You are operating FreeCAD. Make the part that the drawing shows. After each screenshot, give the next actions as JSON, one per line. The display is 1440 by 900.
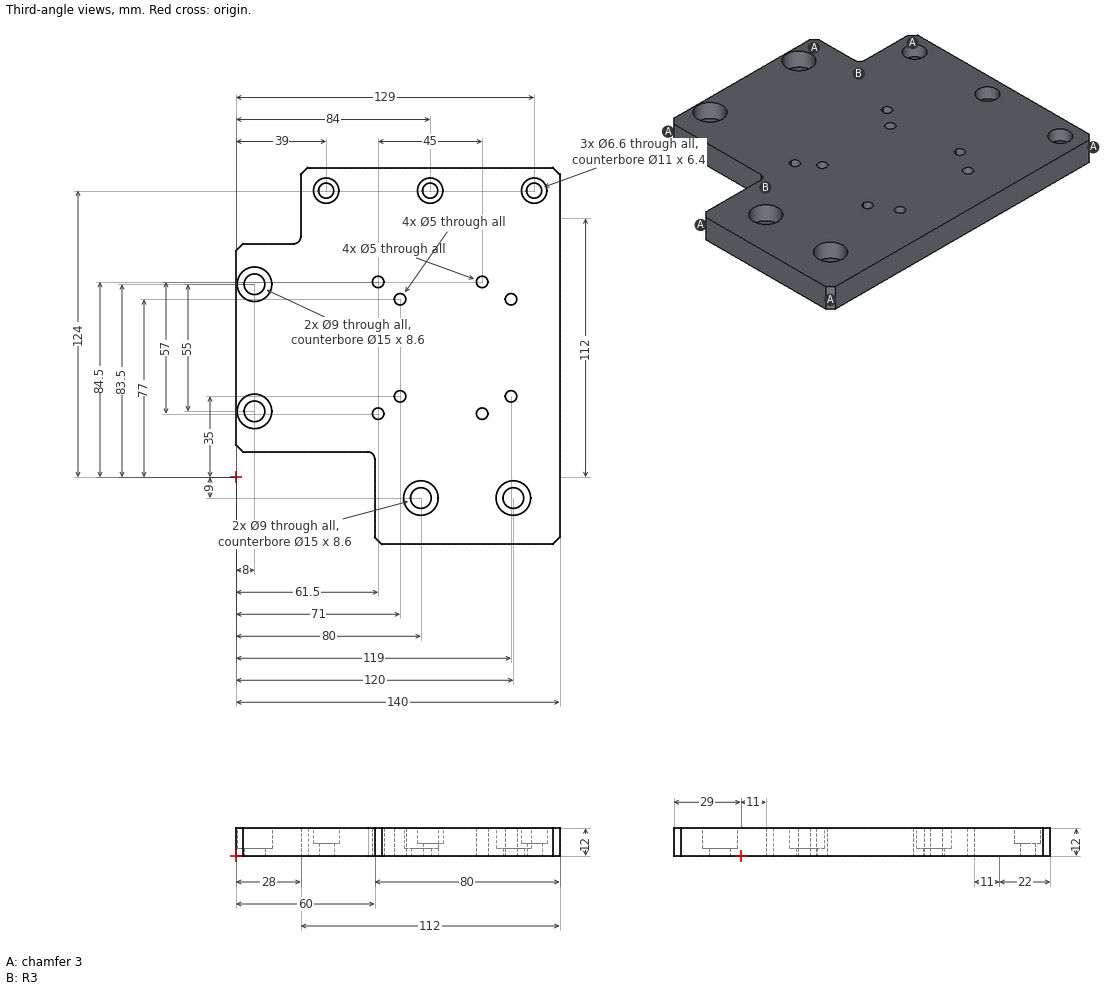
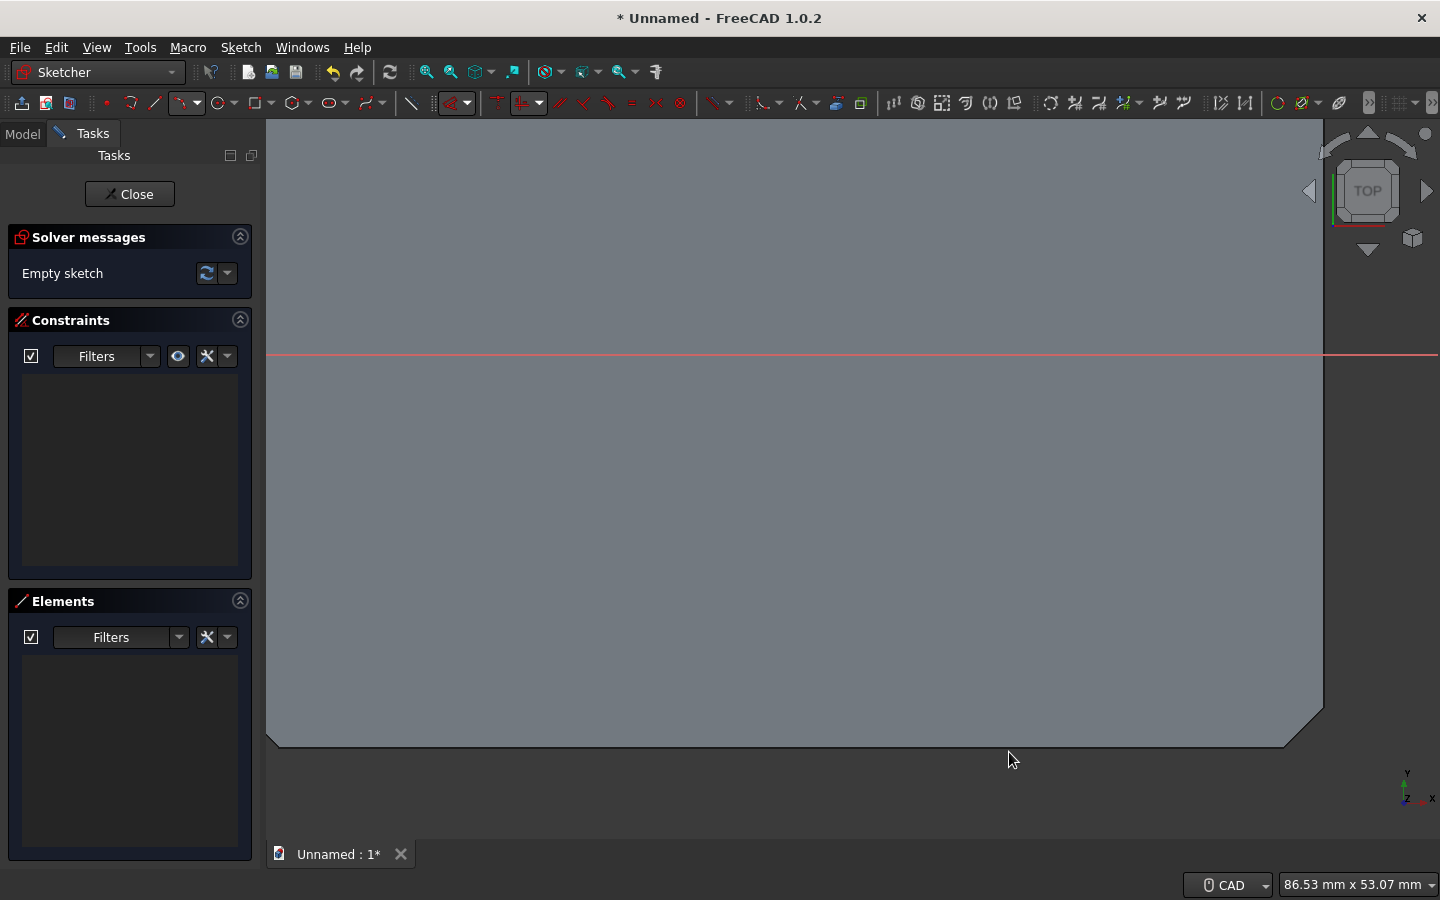
{"action": "key", "text": "g c"}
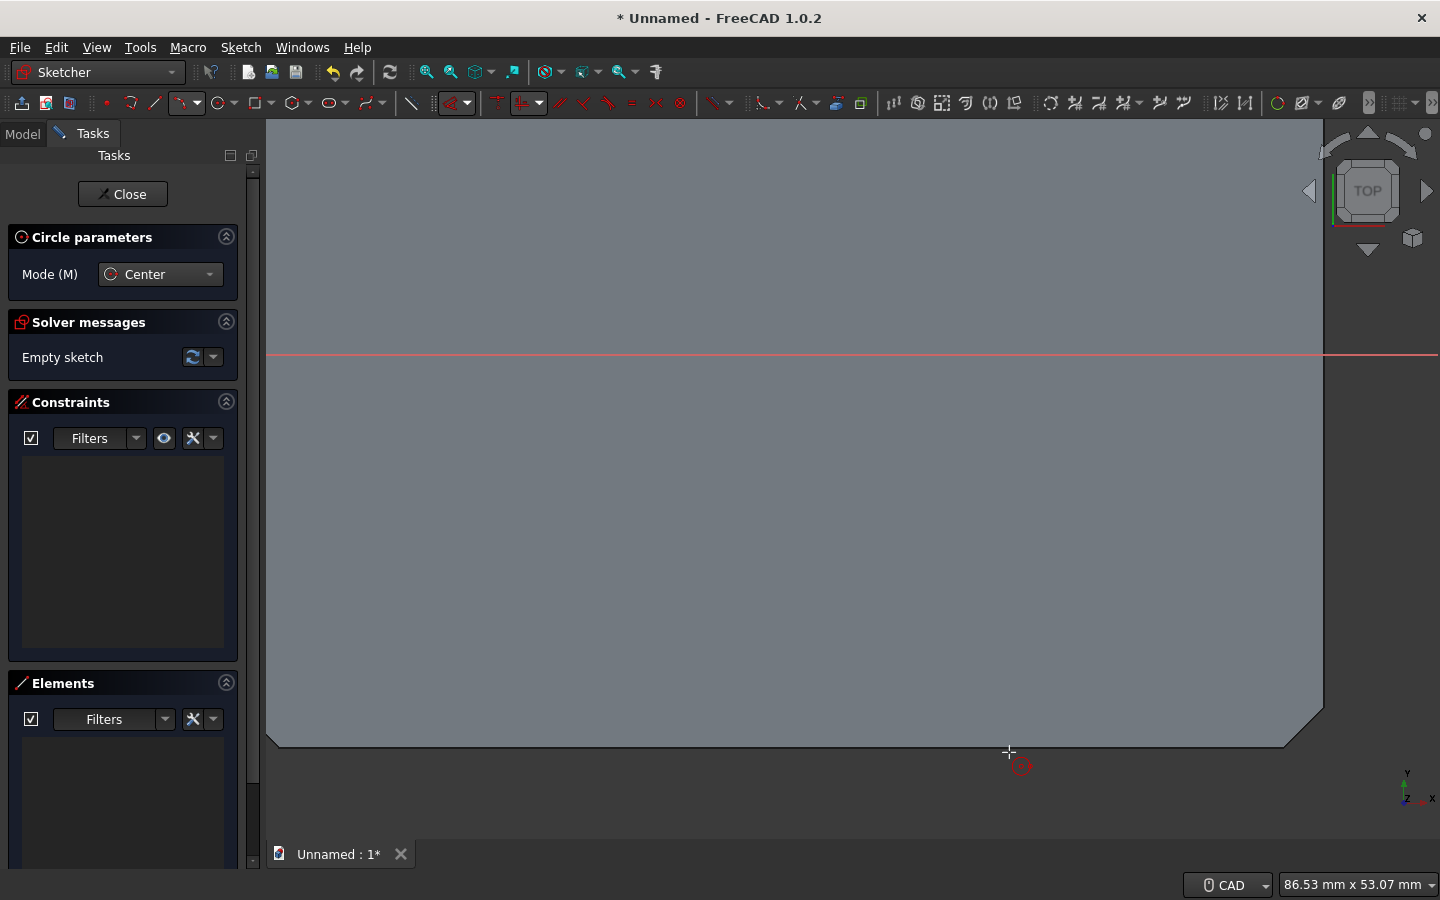
{"action": "left_click", "coordinate": [510, 477]}
{"action": "mouse_move", "coordinate": [553, 433]}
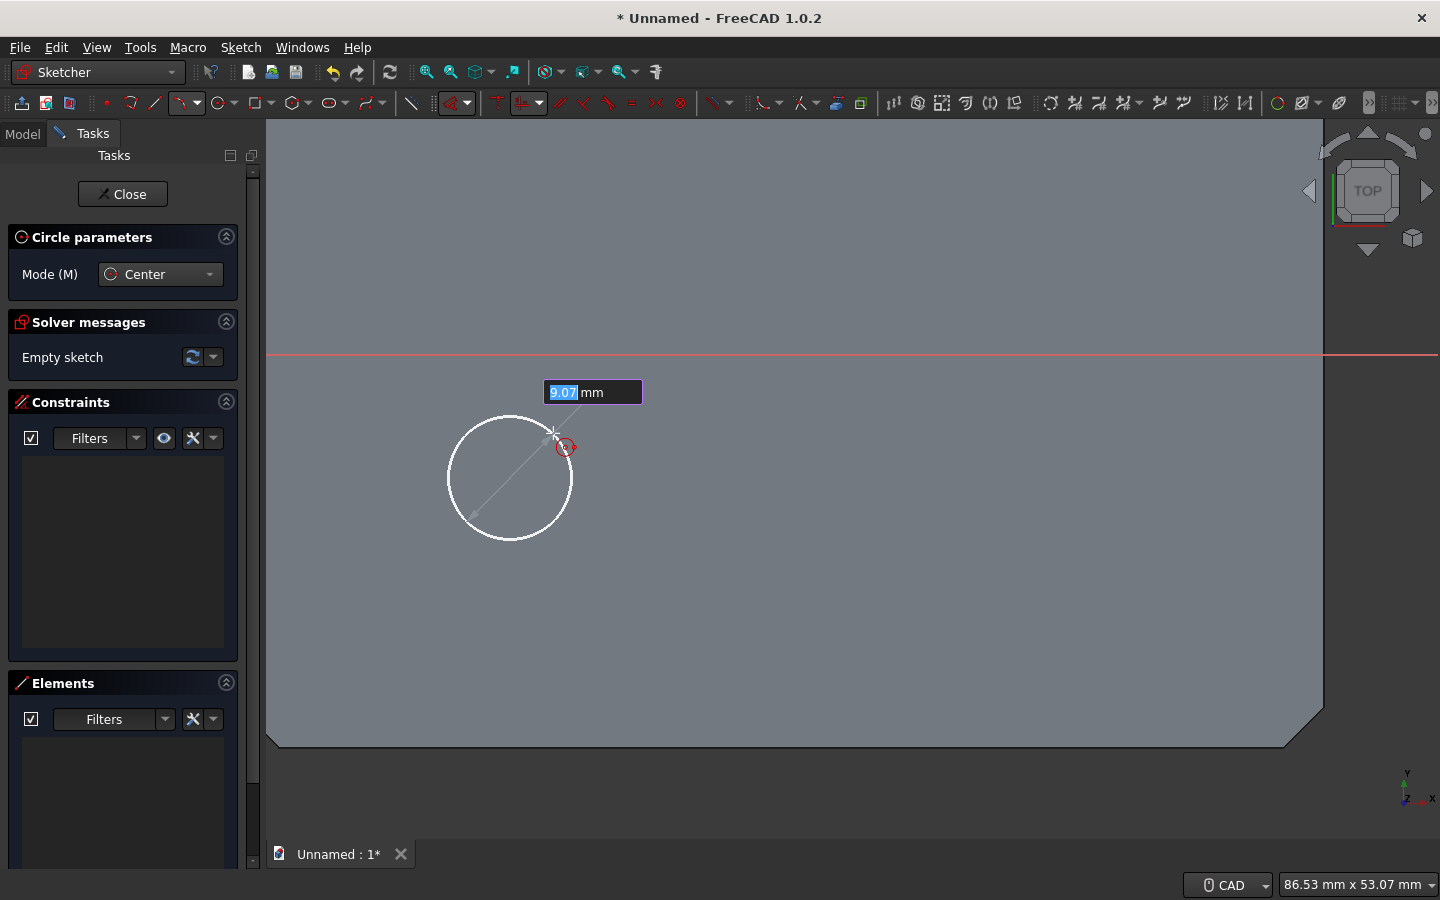
{"action": "type", "text": "9"}
{"action": "key", "text": "Return"}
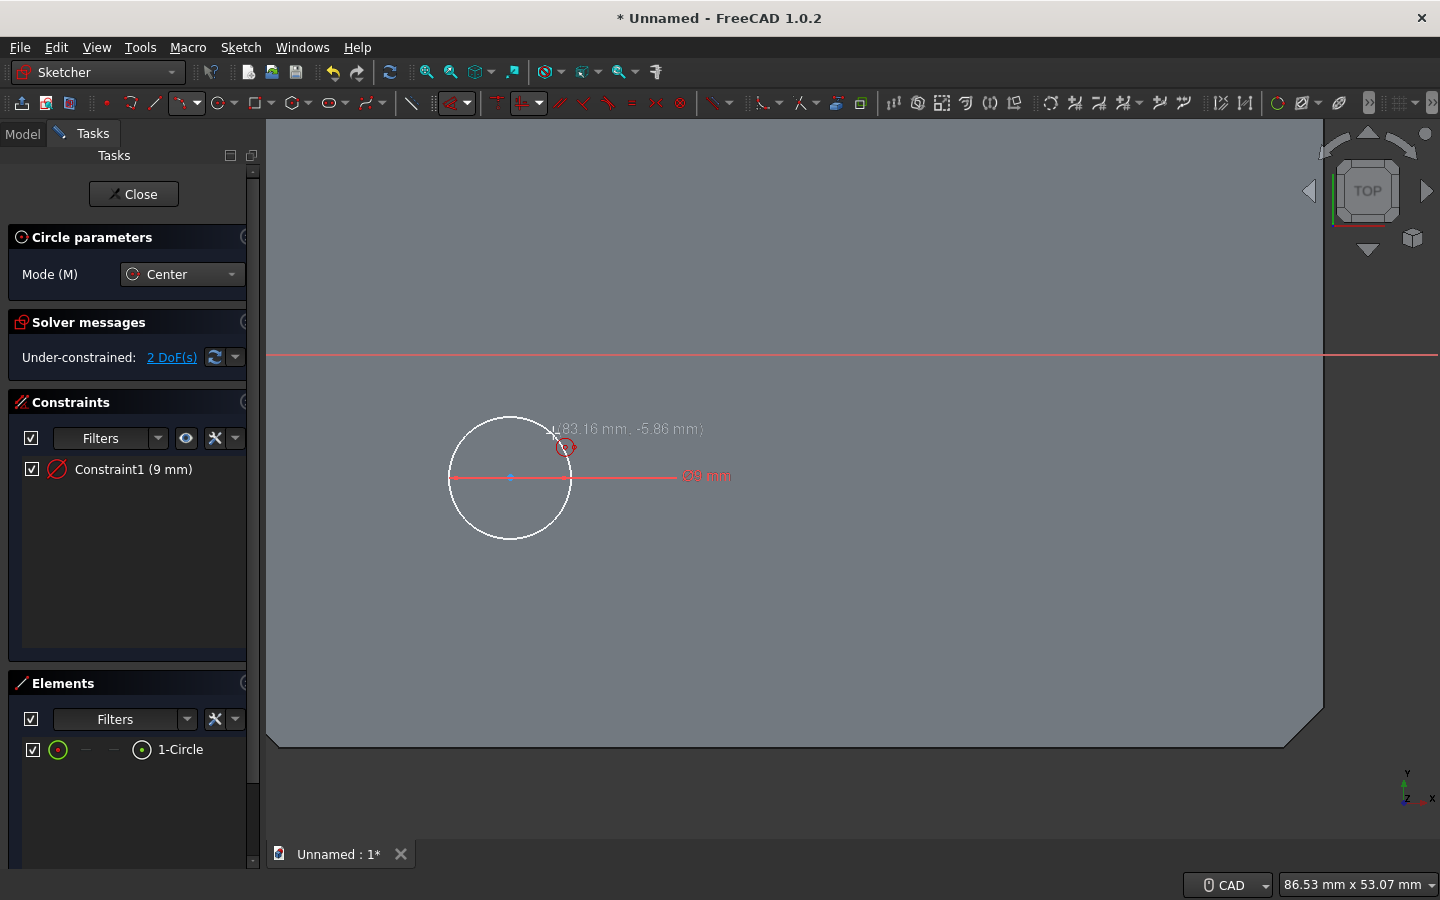
{"action": "left_click", "coordinate": [1053, 477]}
{"action": "mouse_move", "coordinate": [1096, 433]}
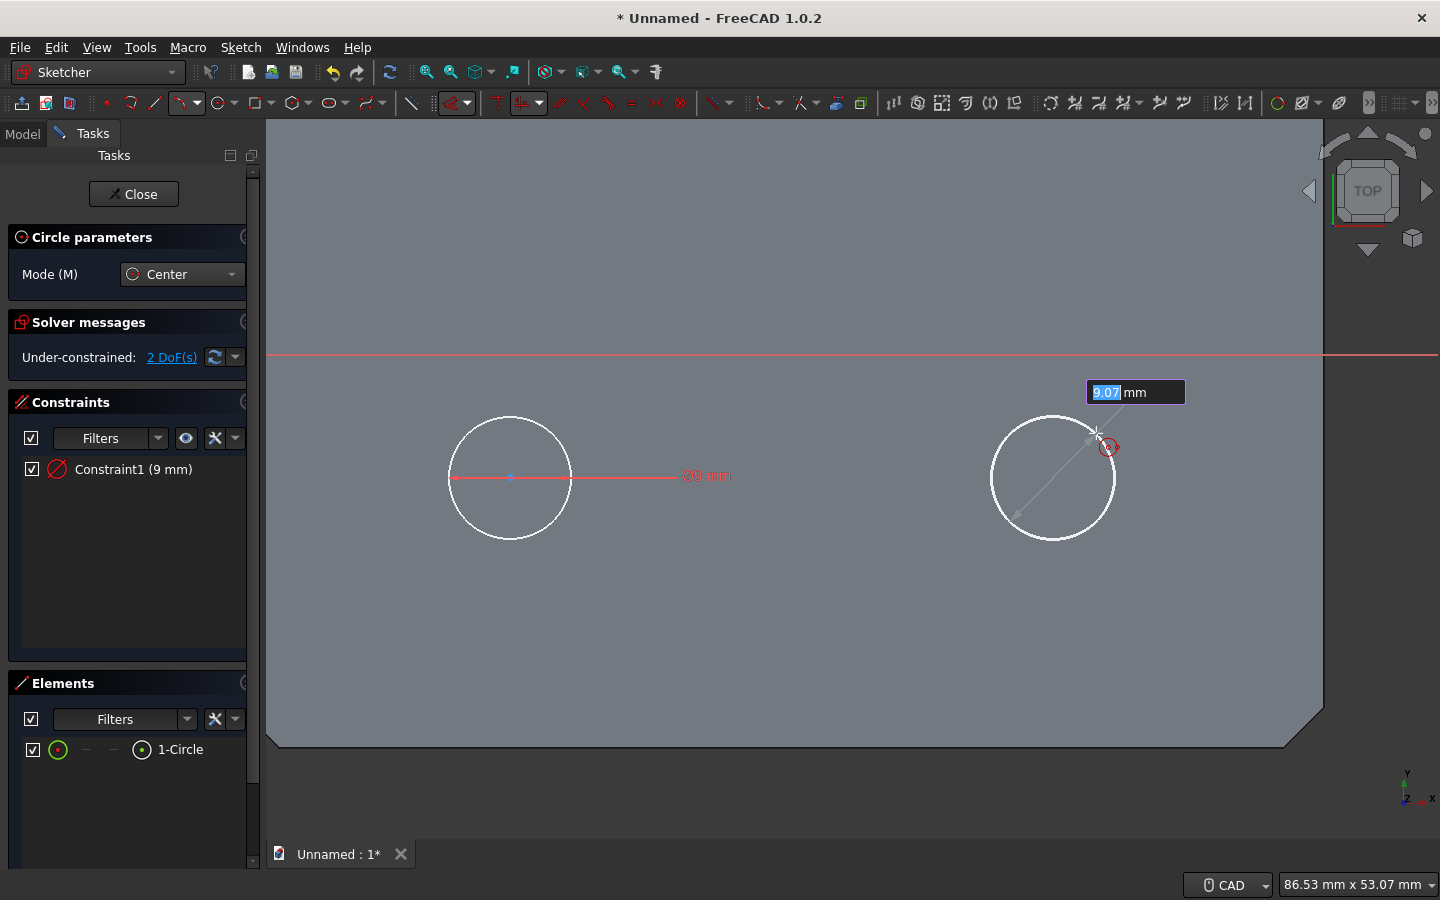
{"action": "type", "text": "9"}
{"action": "key", "text": "Return"}
{"action": "key", "text": "Escape"}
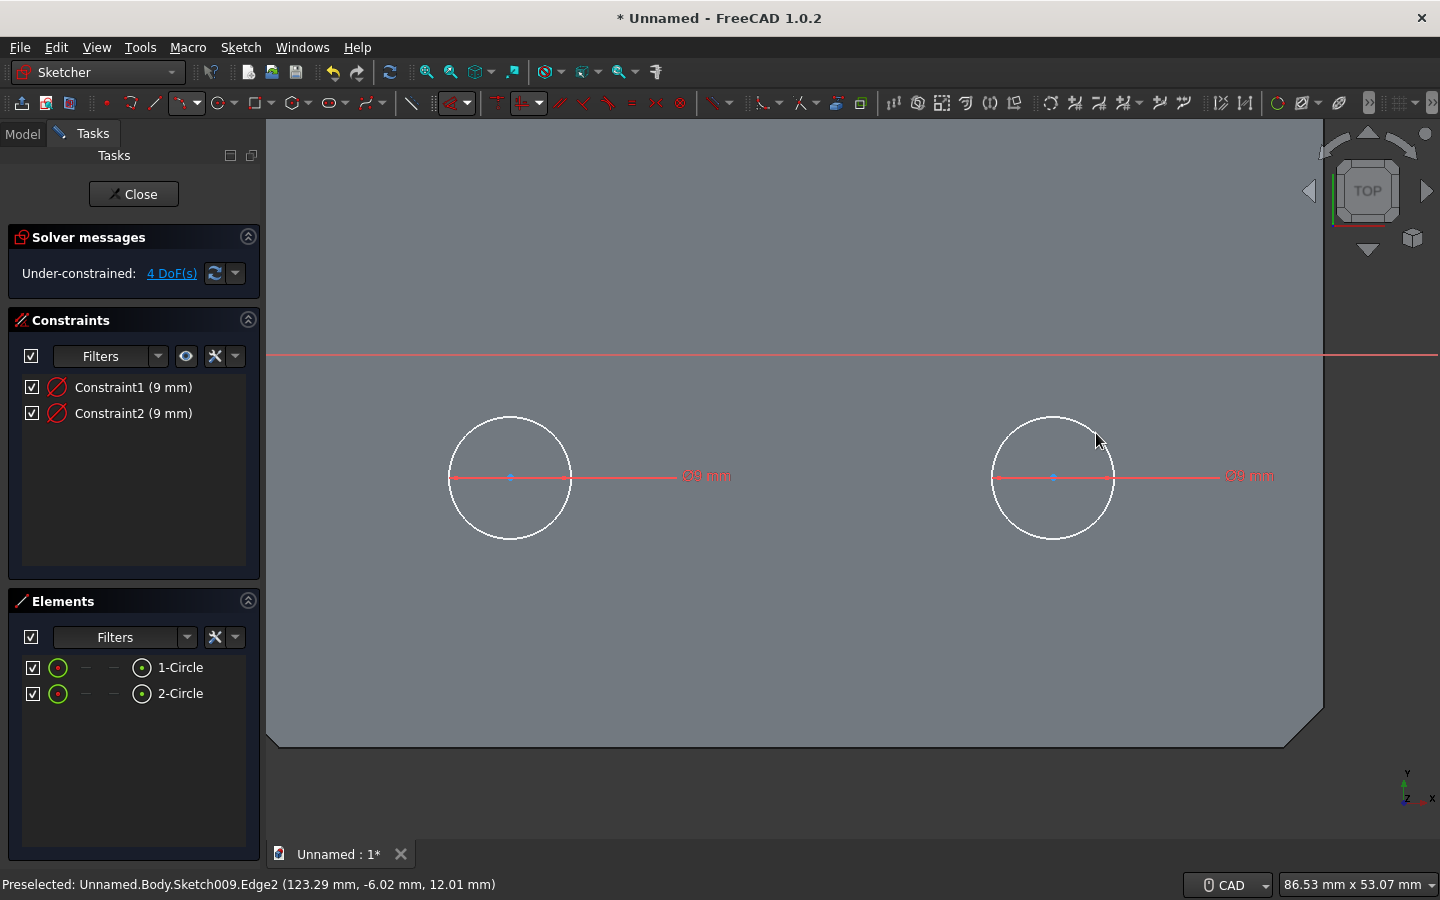
{"action": "left_click", "coordinate": [510, 478]}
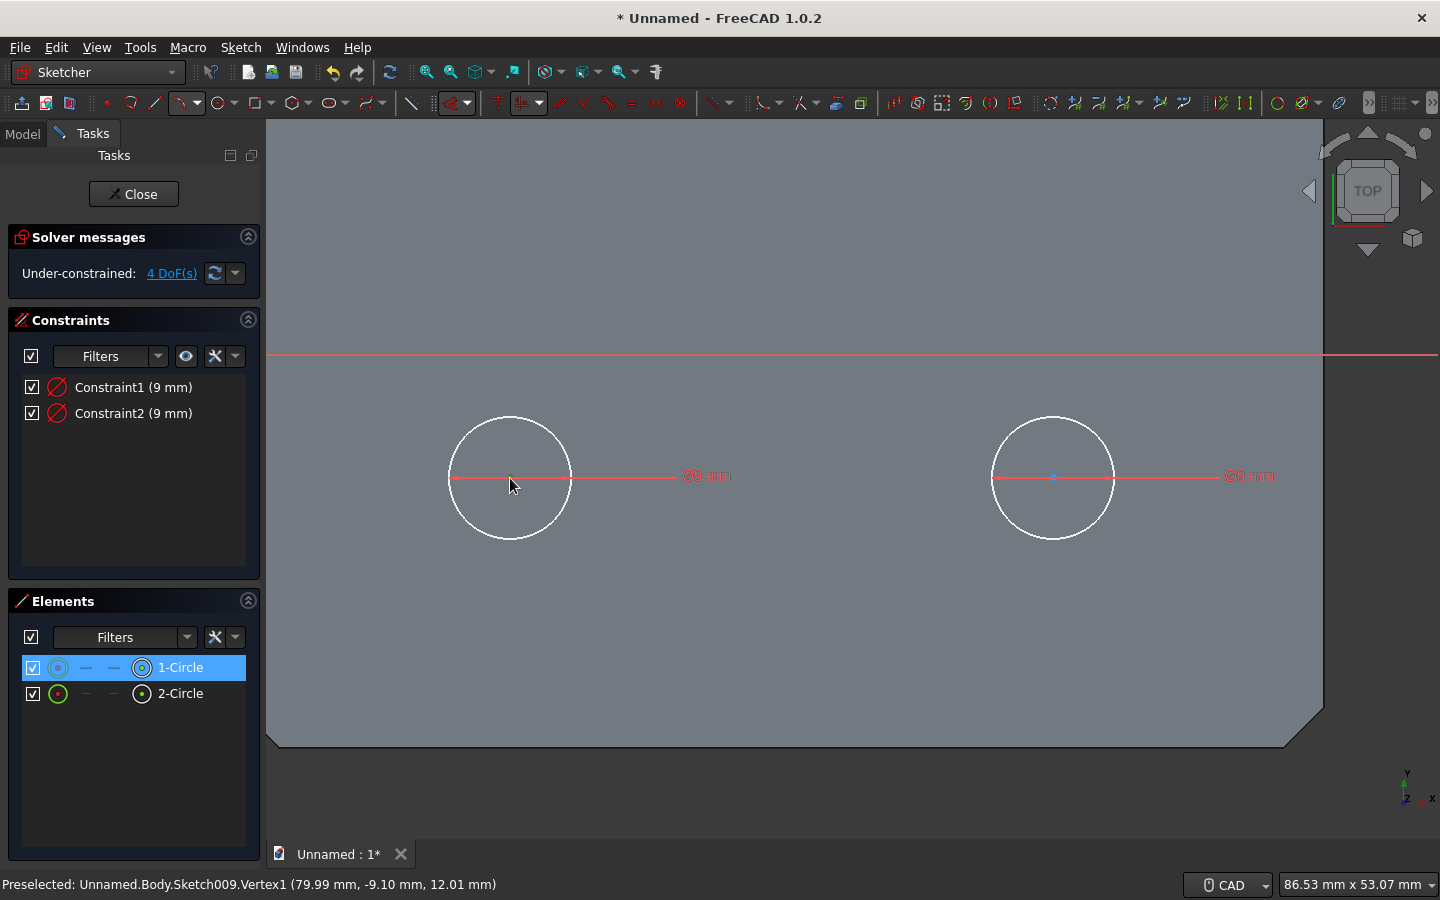
{"action": "key", "text": "i"}